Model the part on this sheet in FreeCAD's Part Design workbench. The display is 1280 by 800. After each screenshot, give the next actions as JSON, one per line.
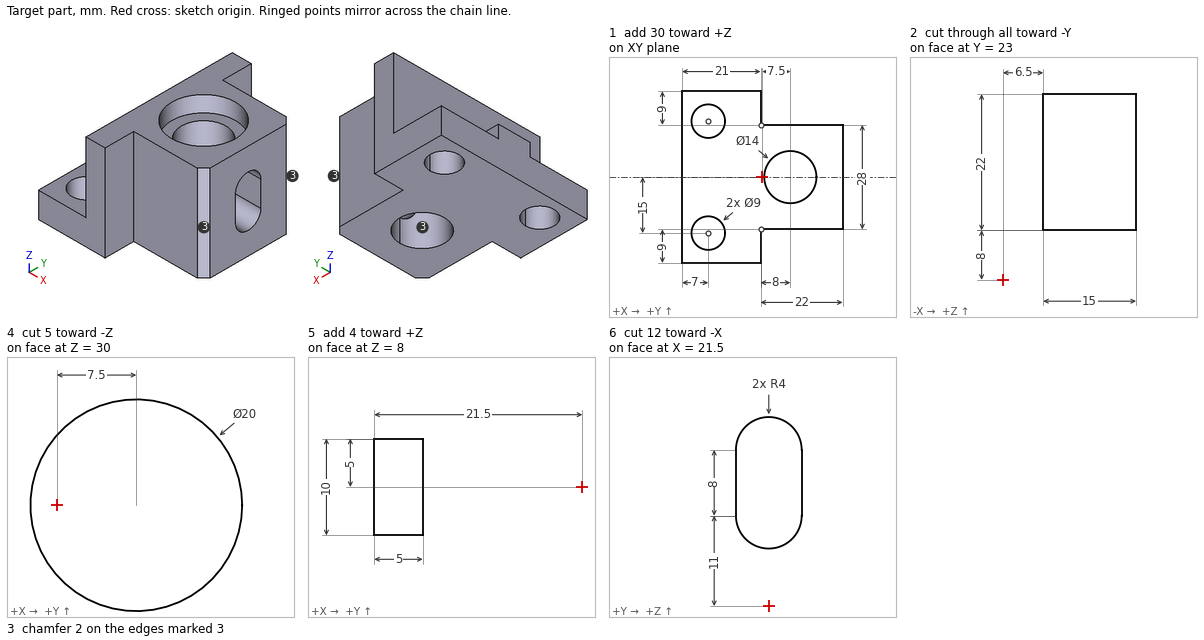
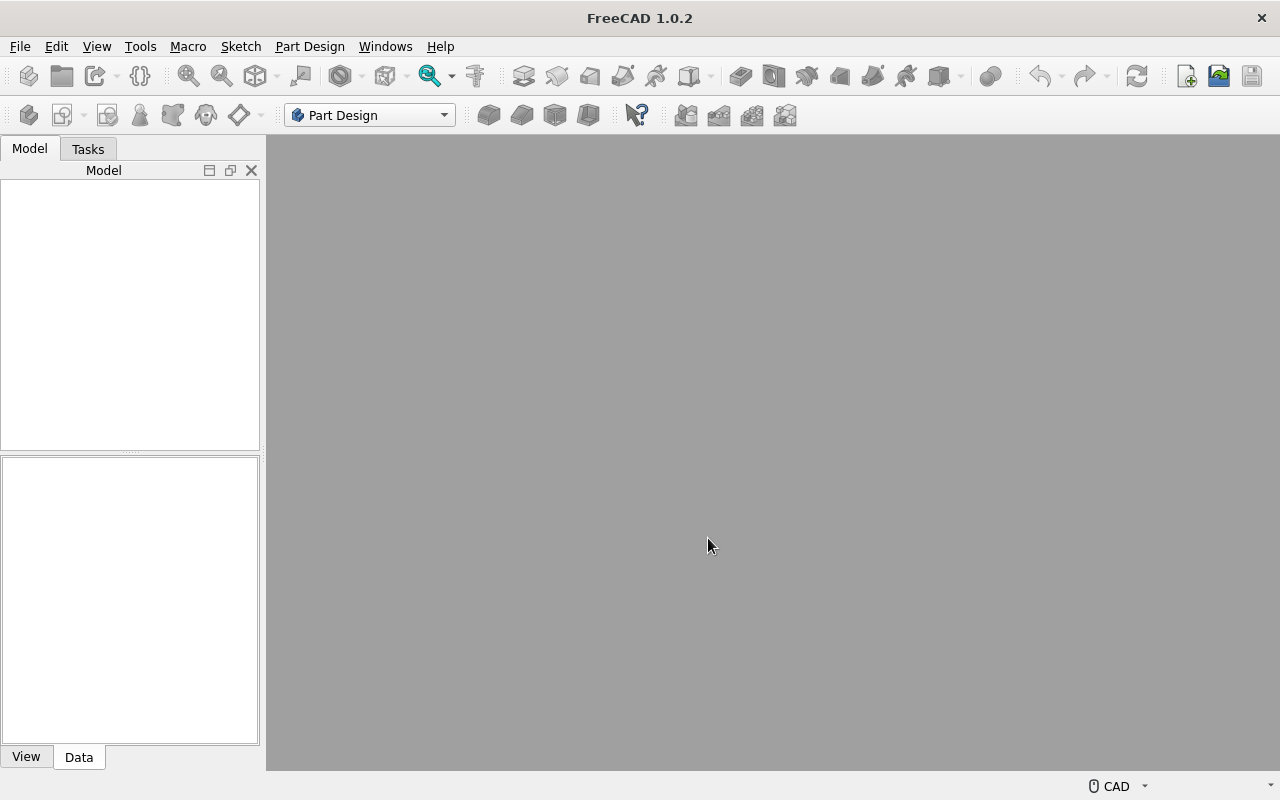
{"action": "key", "text": "ctrl+n"}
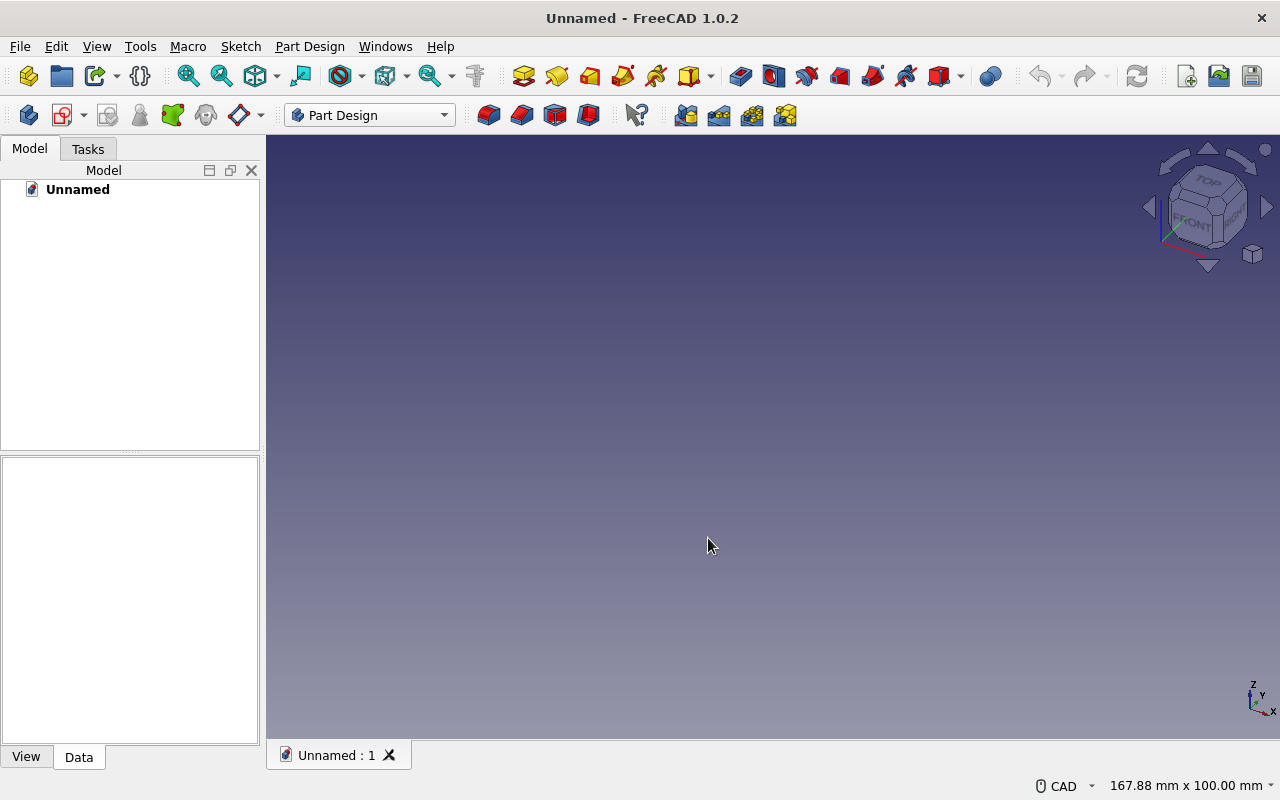
{"action": "left_click", "coordinate": [62, 116]}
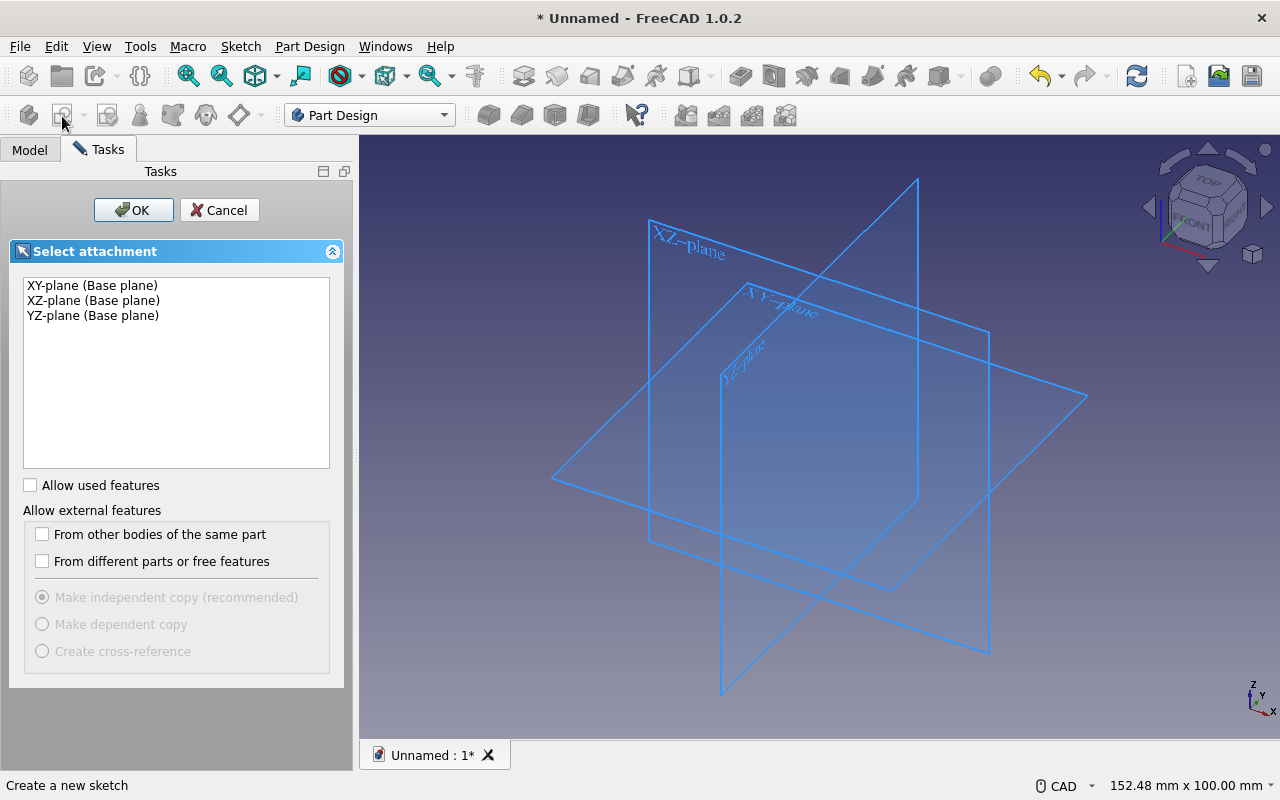
{"action": "left_click", "coordinate": [84, 286]}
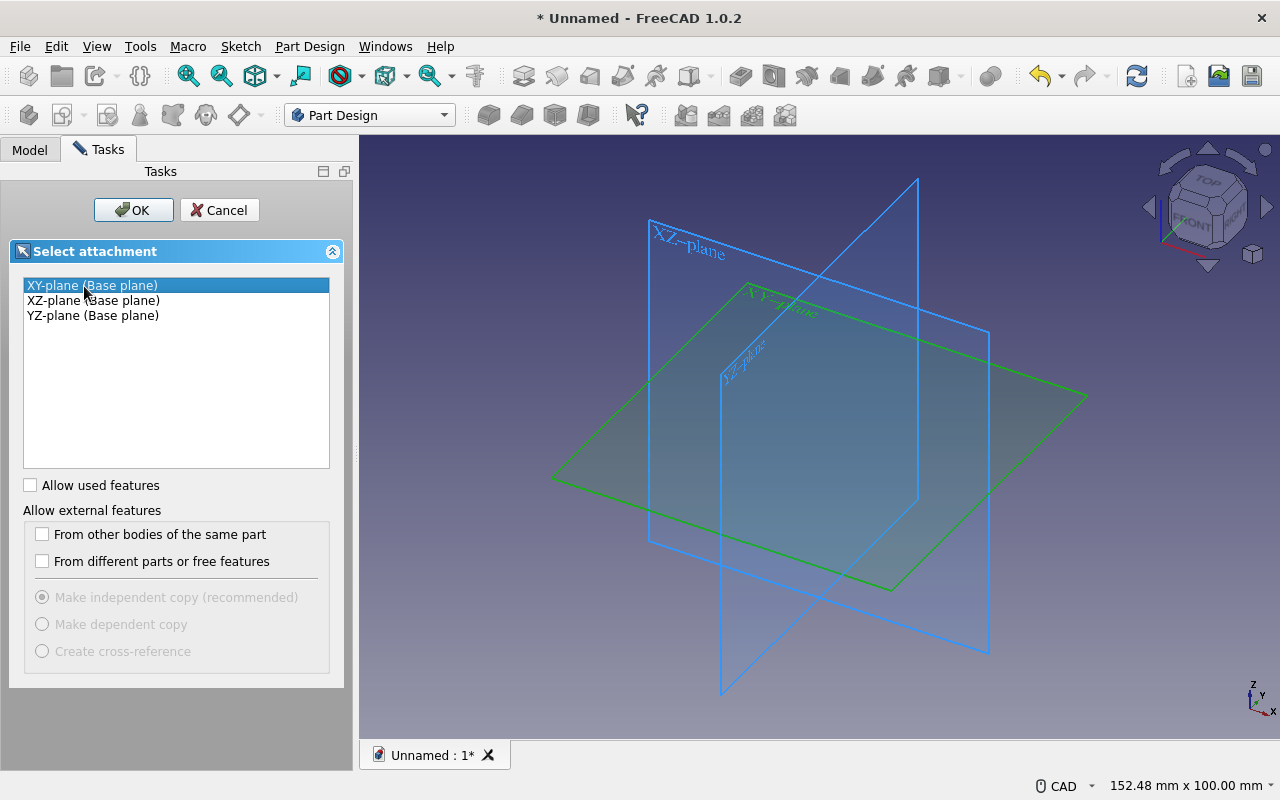
{"action": "left_click", "coordinate": [134, 210]}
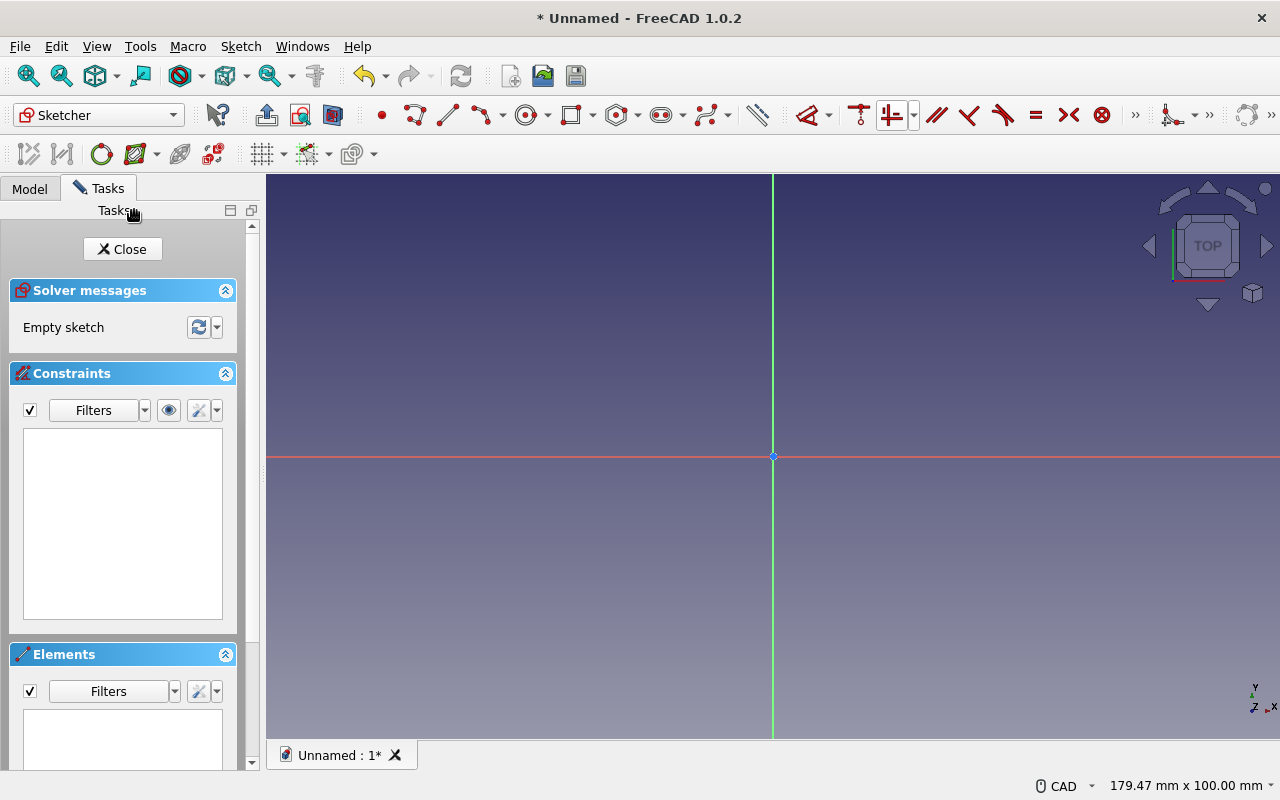
{"action": "scroll", "coordinate": [912, 456], "scroll_direction": "up", "scroll_amount": 2}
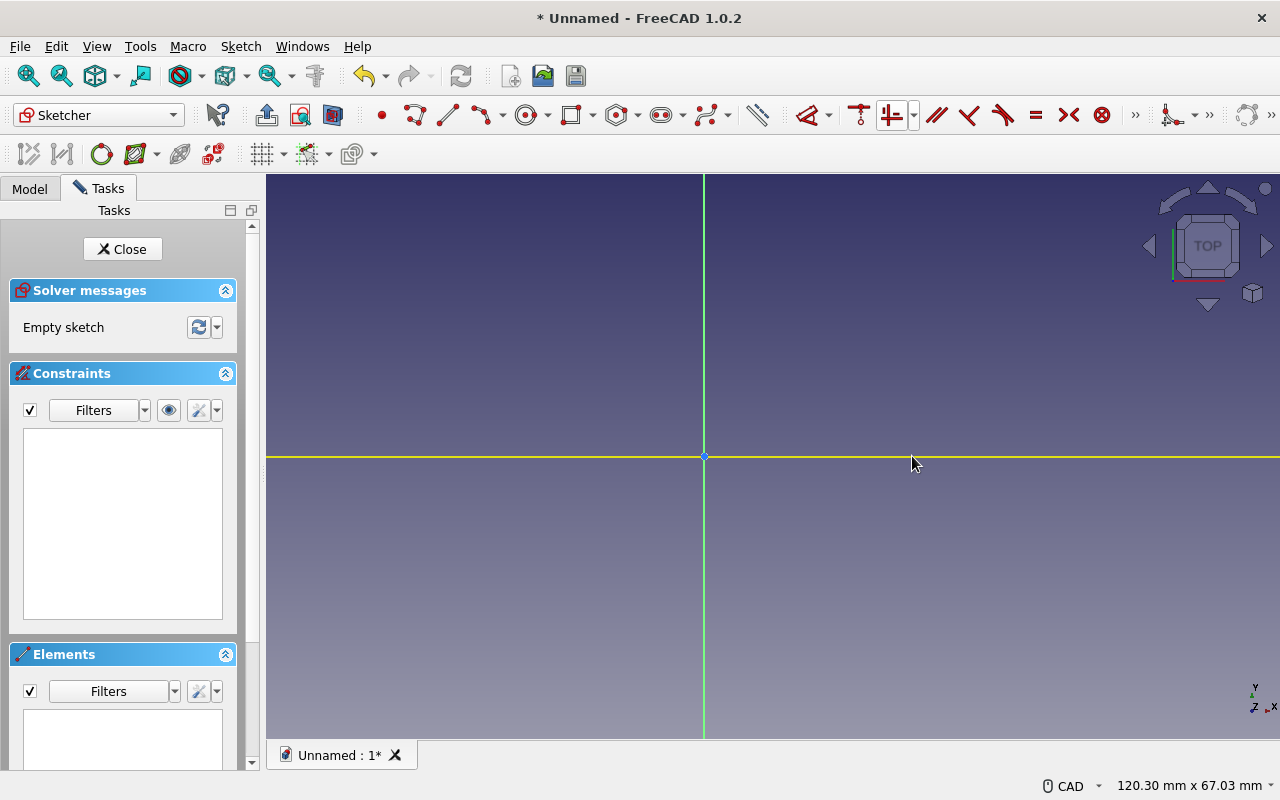
{"action": "key", "text": "g m"}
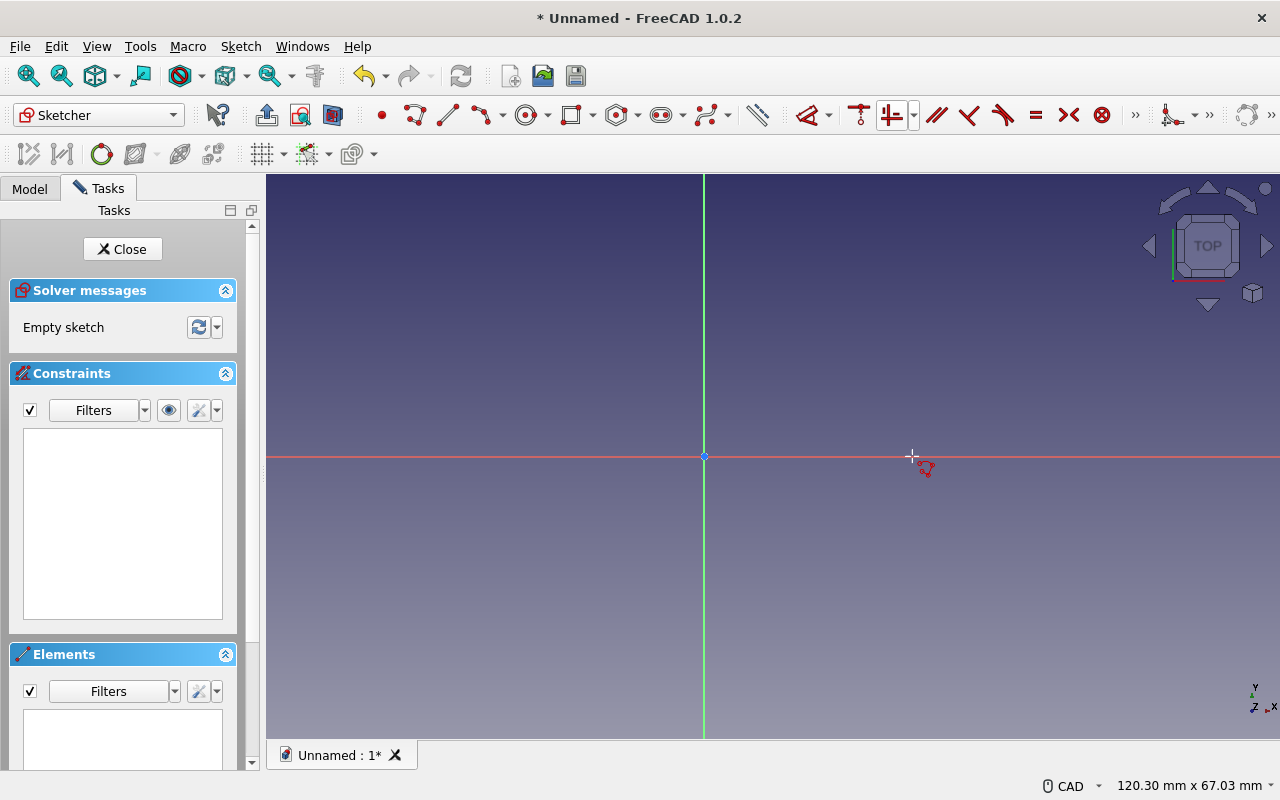
{"action": "scroll", "coordinate": [700, 575], "scroll_direction": "up", "scroll_amount": 7}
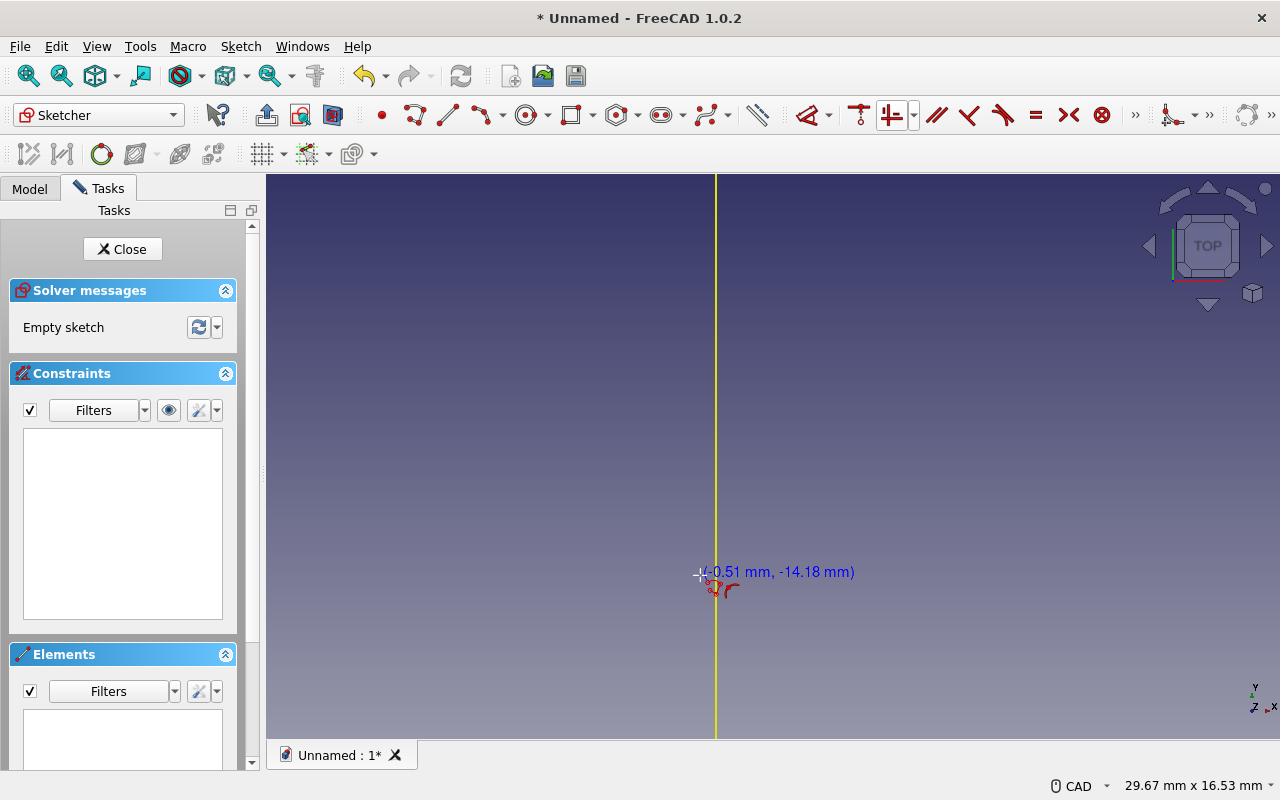
{"action": "left_click", "coordinate": [699, 571]}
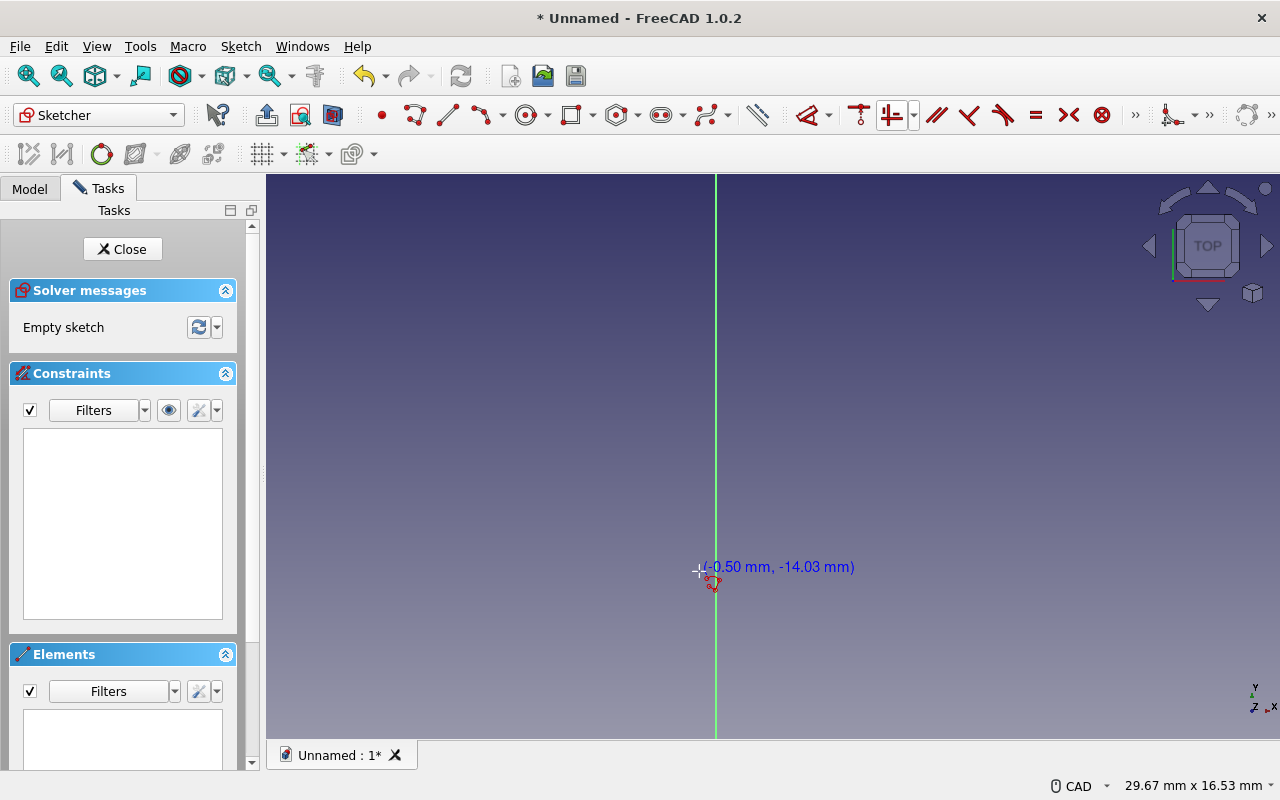
{"action": "scroll", "coordinate": [701, 576], "scroll_direction": "down", "scroll_amount": 7}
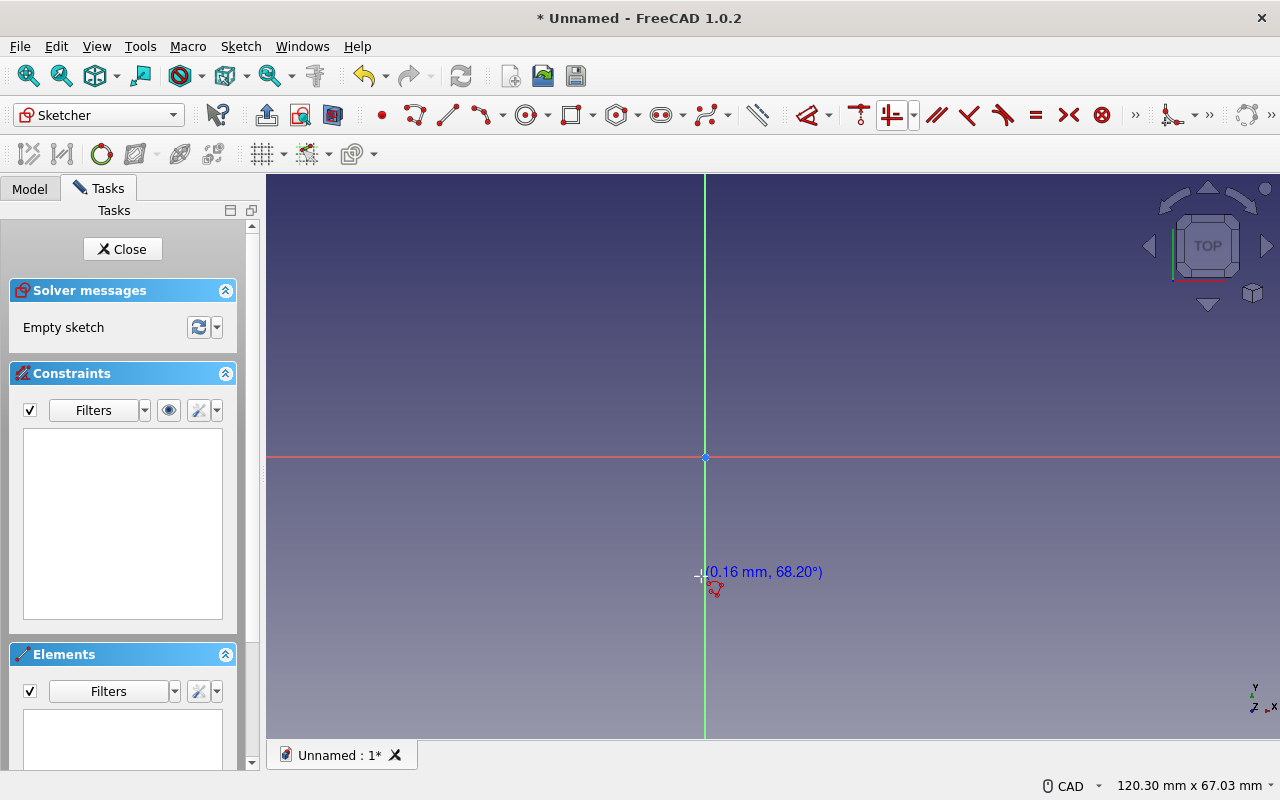
{"action": "left_click", "coordinate": [886, 575]}
{"action": "left_click", "coordinate": [886, 339]}